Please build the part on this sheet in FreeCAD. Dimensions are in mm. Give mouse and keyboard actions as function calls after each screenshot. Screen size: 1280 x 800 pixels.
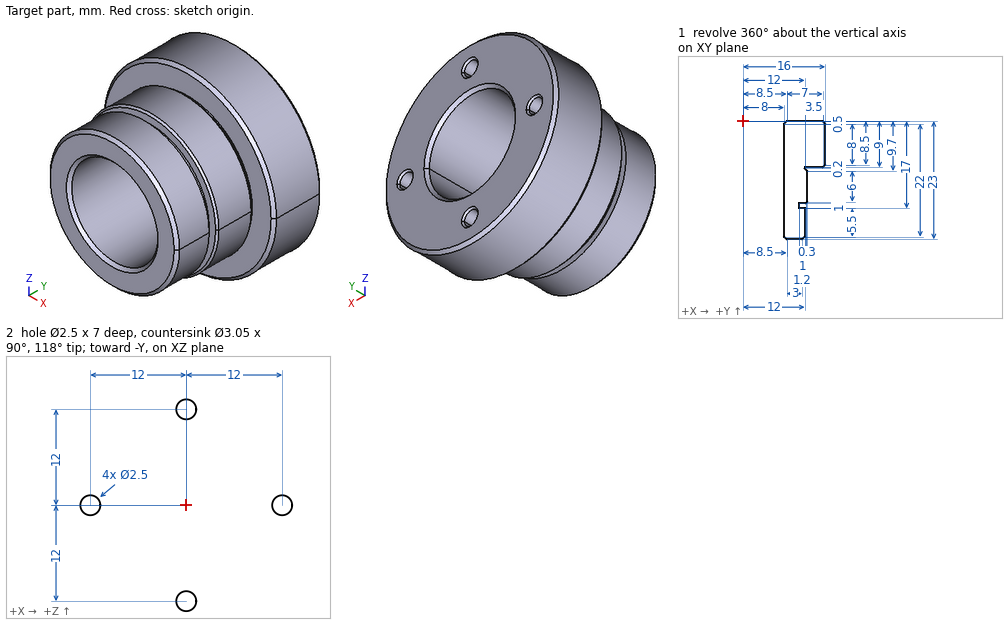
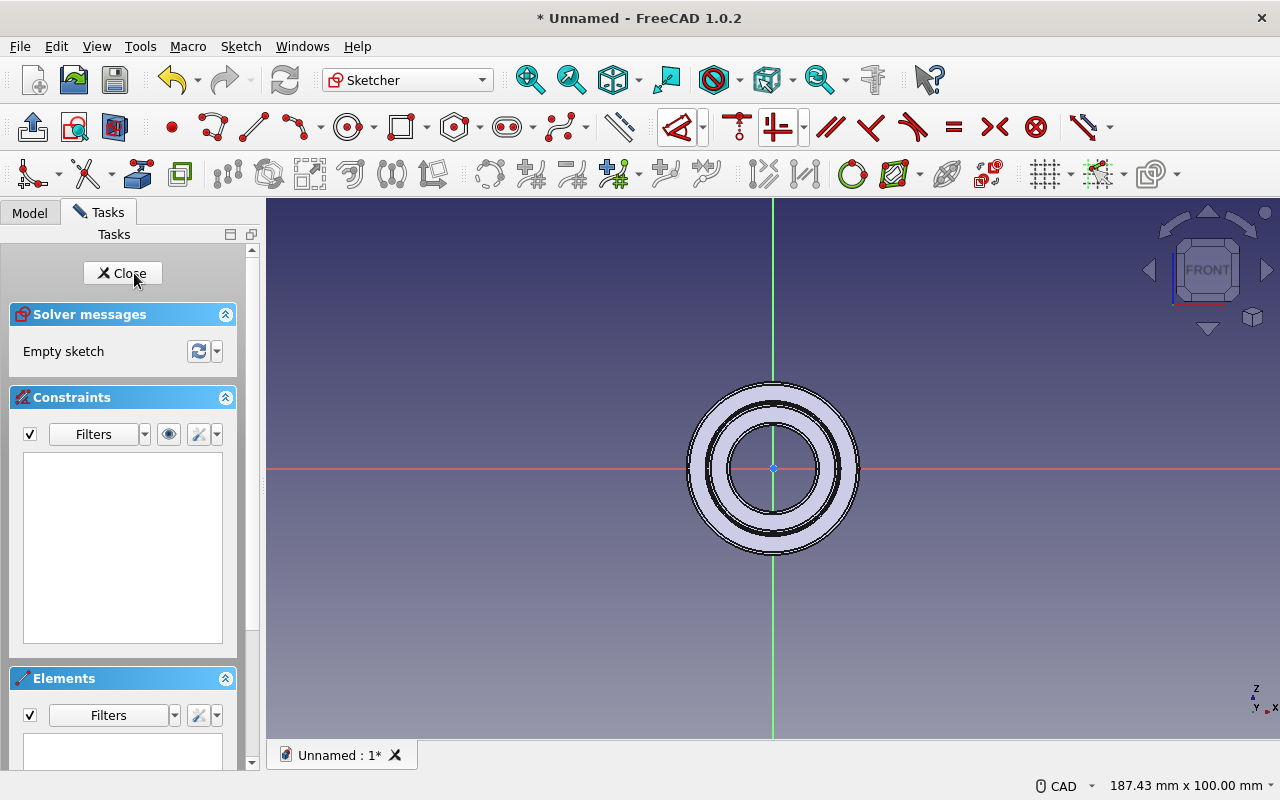
click(115, 128)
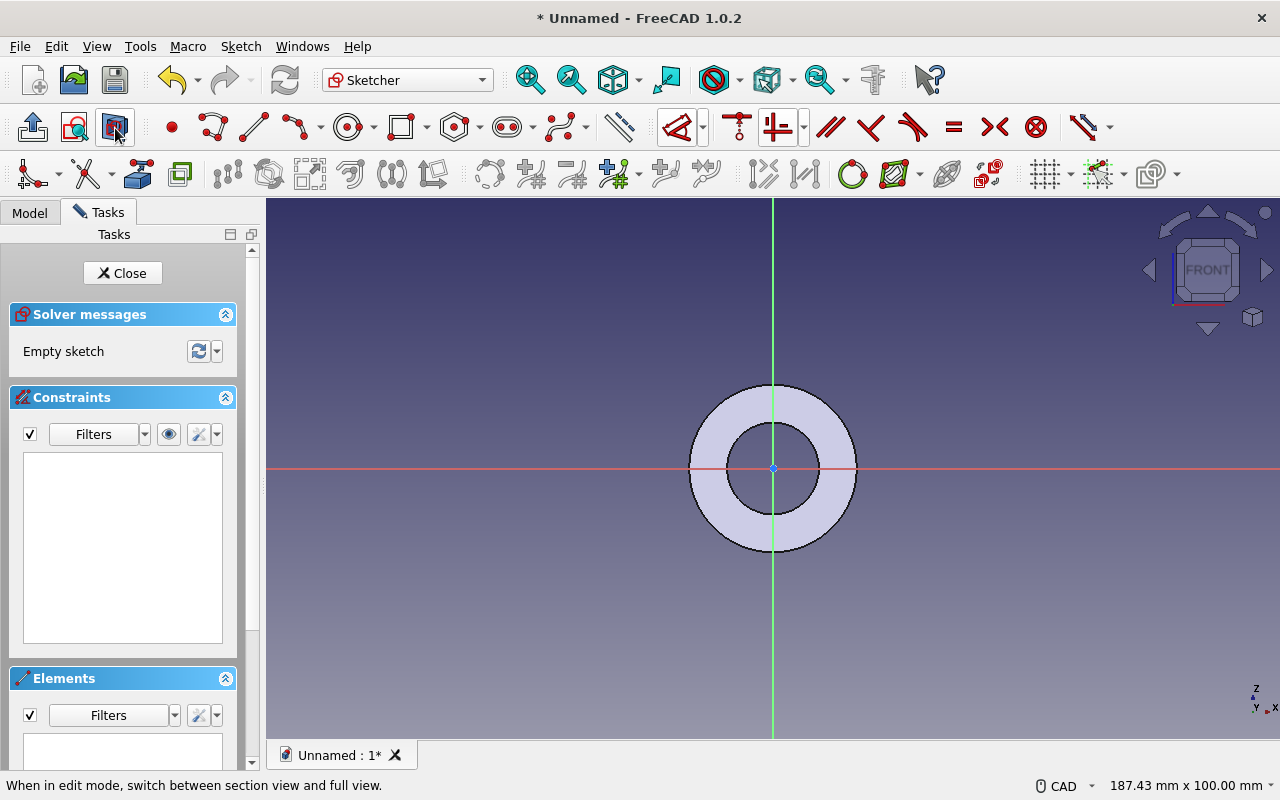
scroll(829, 469, up, 4)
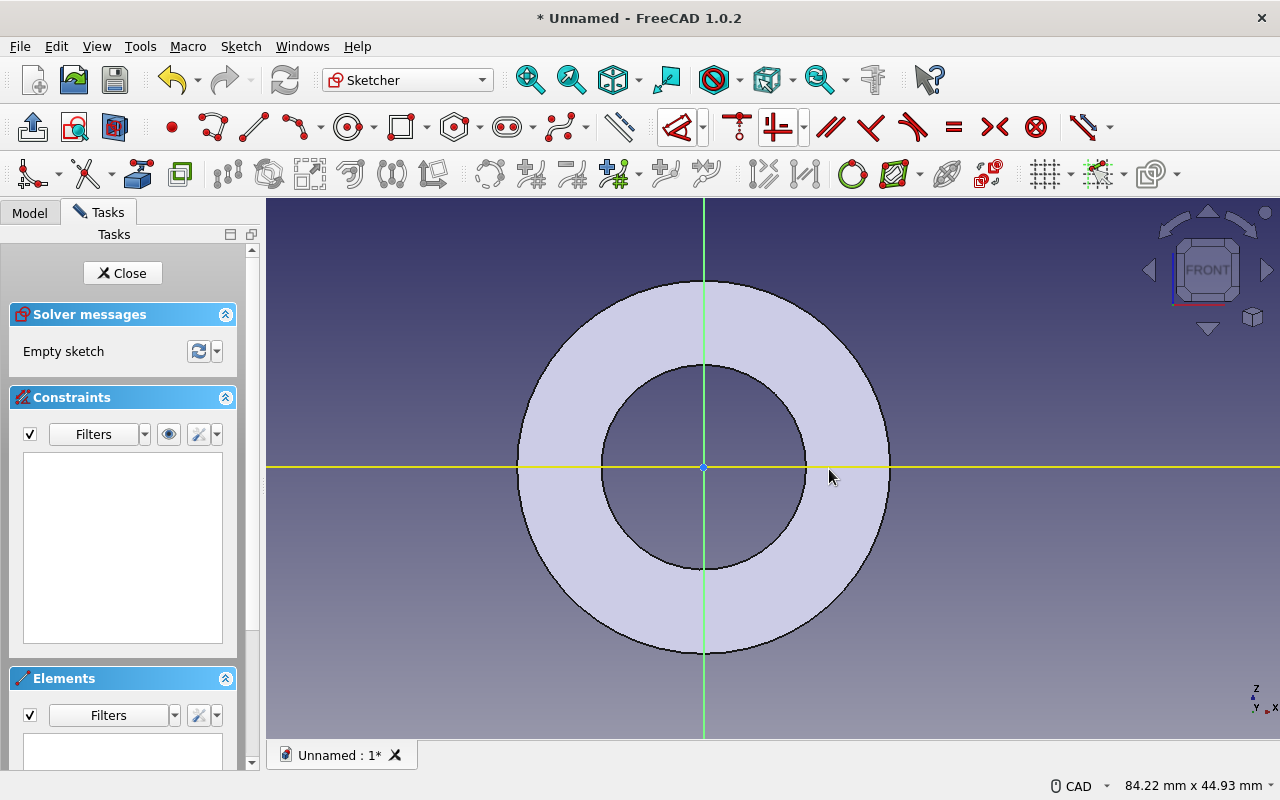
click(348, 128)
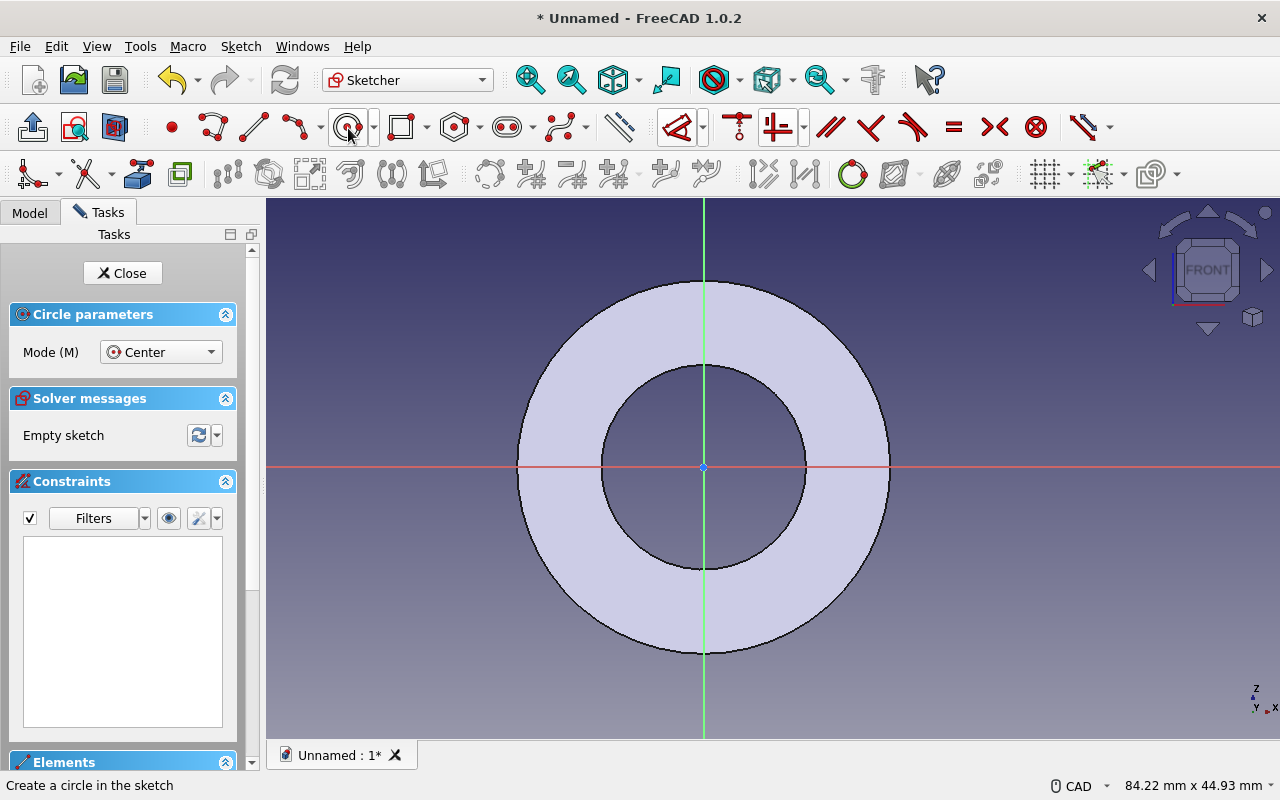
scroll(559, 467, up, 3)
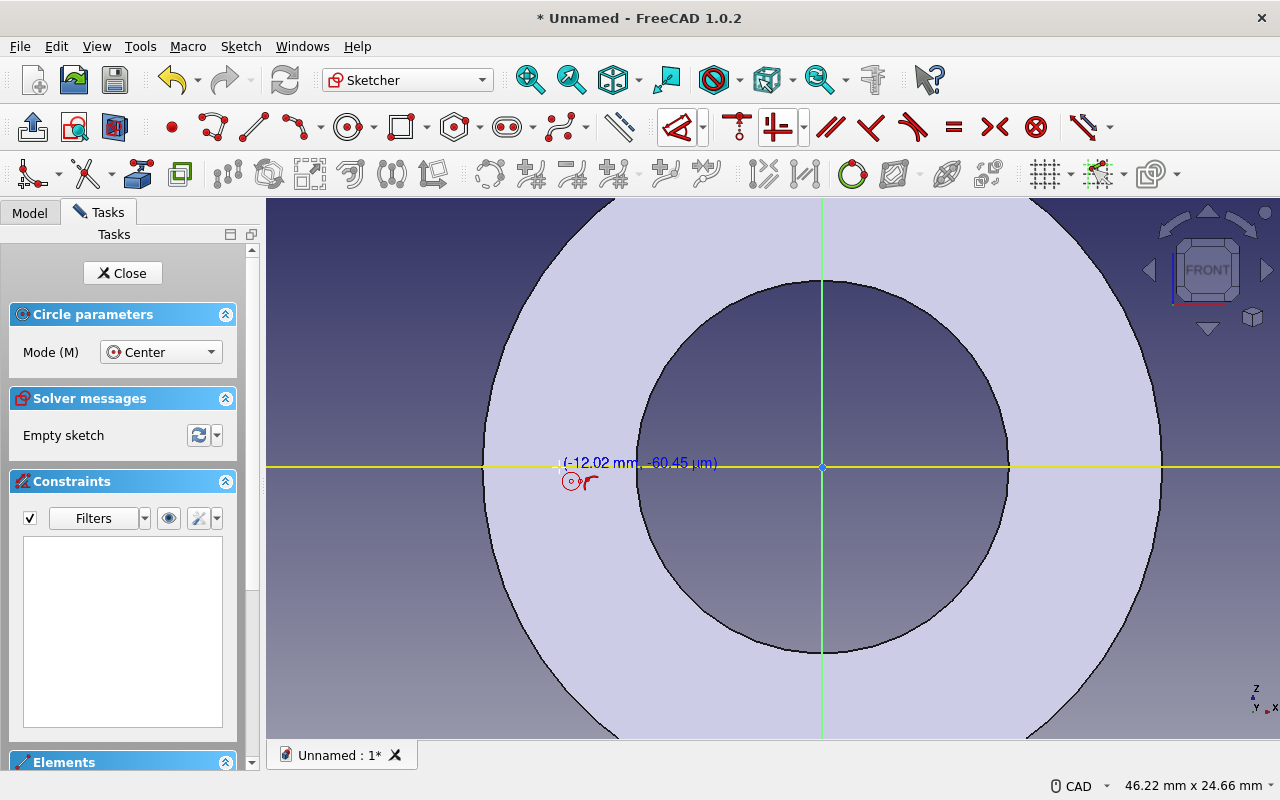
click(559, 467)
click(579, 448)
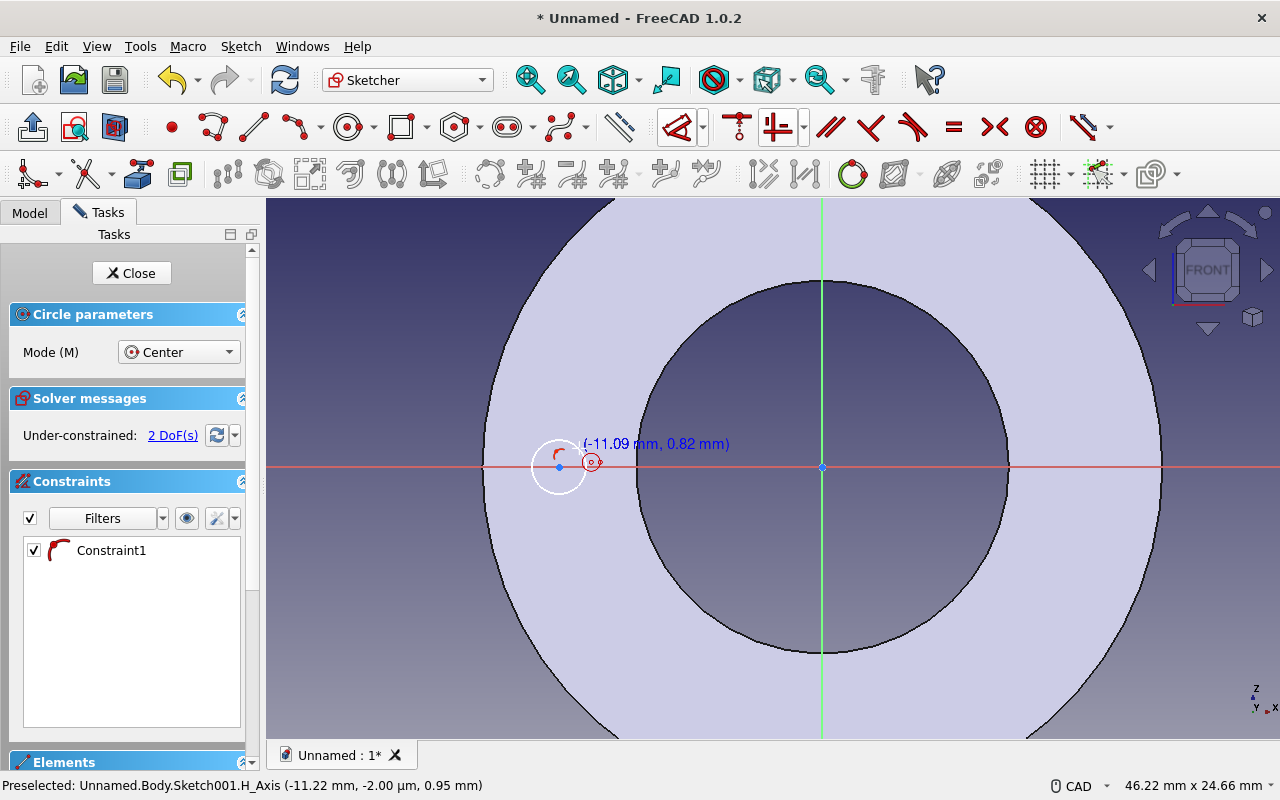
scroll(561, 470, down, 3)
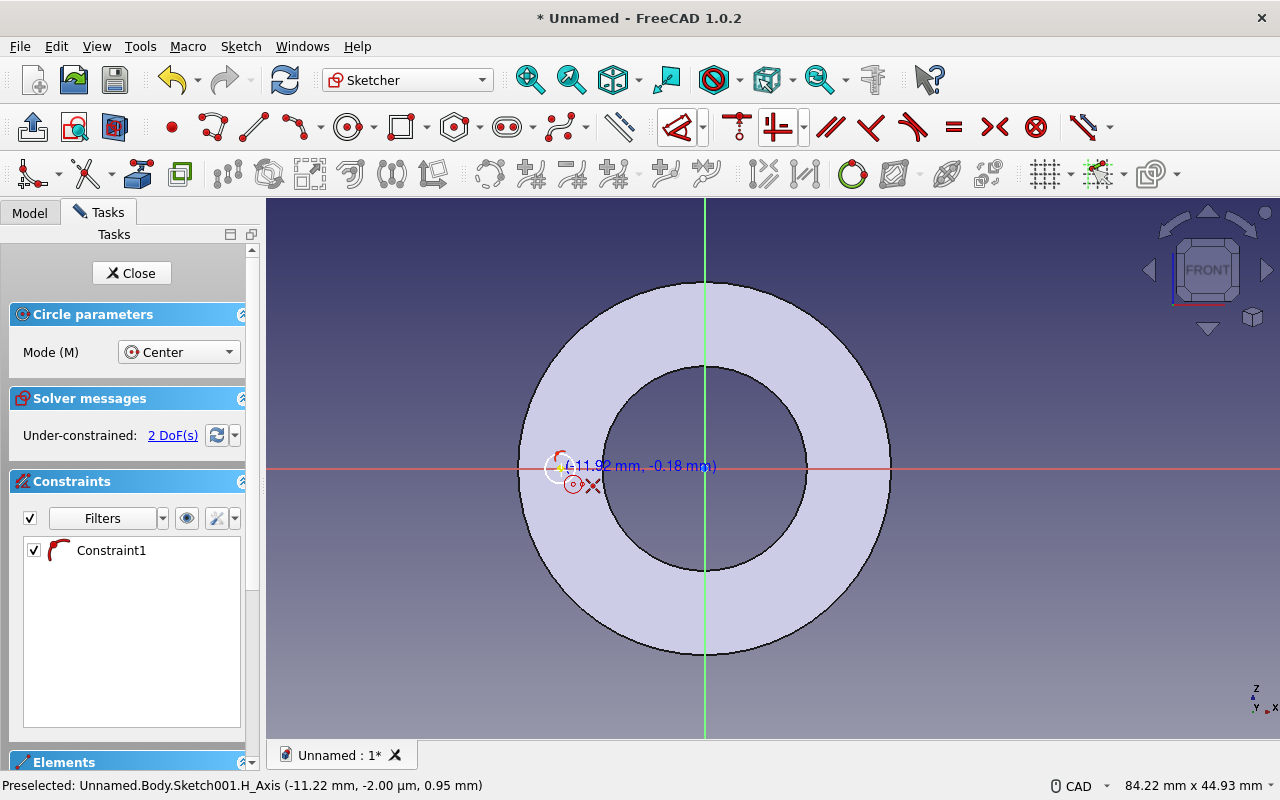
scroll(705, 613, up, 3)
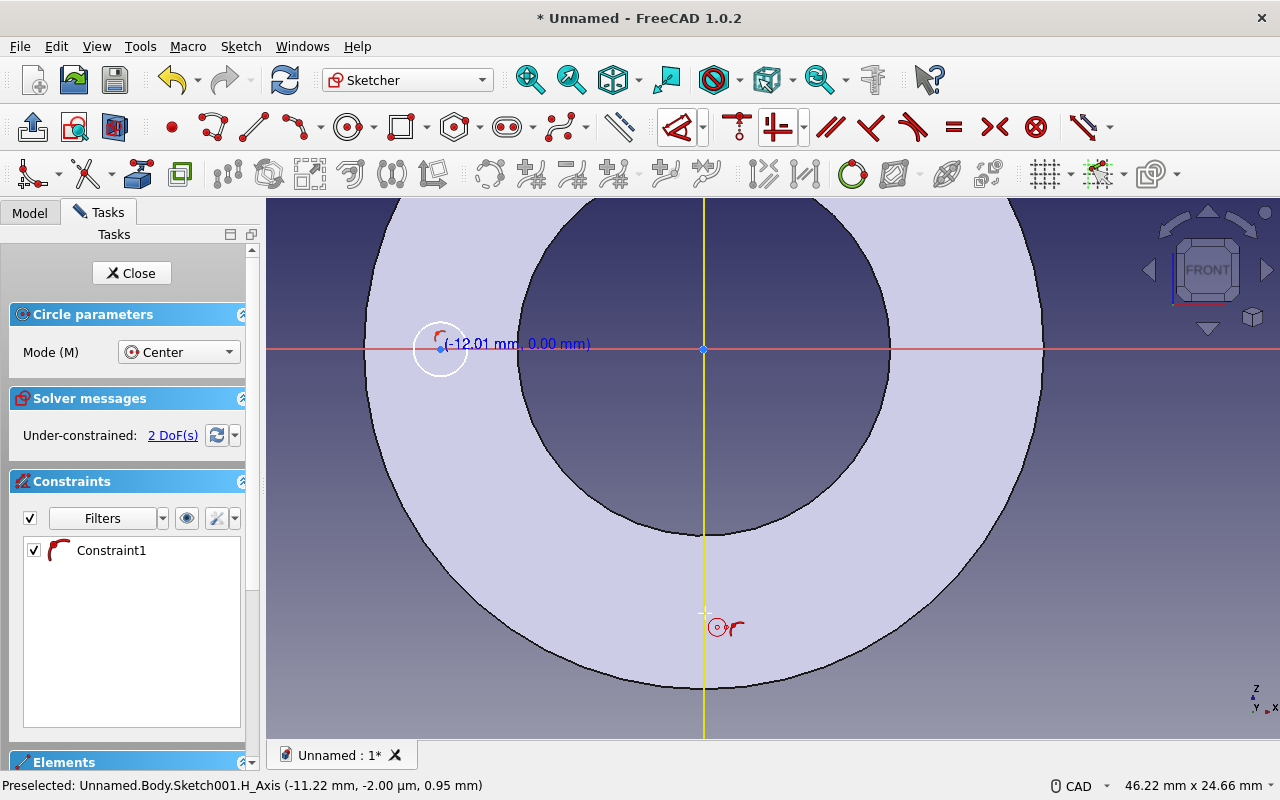
click(704, 613)
click(723, 593)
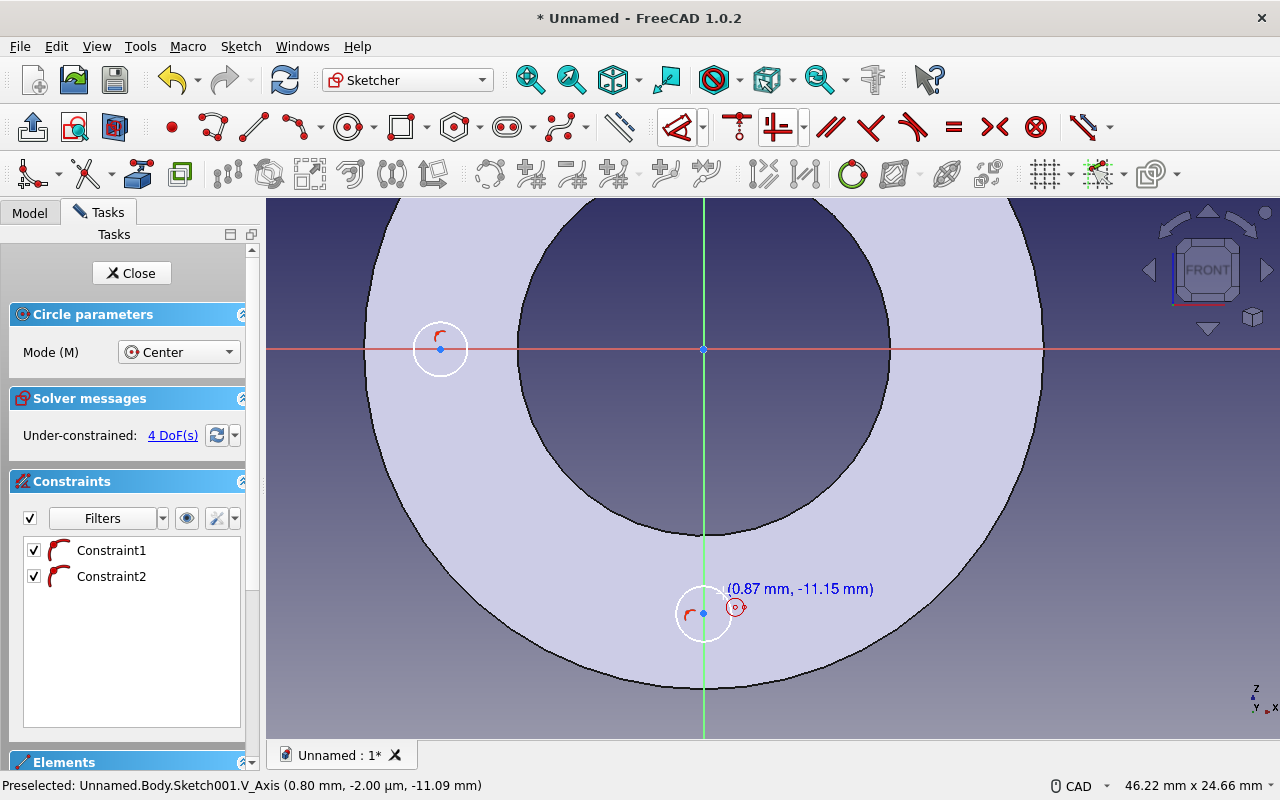
click(967, 349)
click(987, 330)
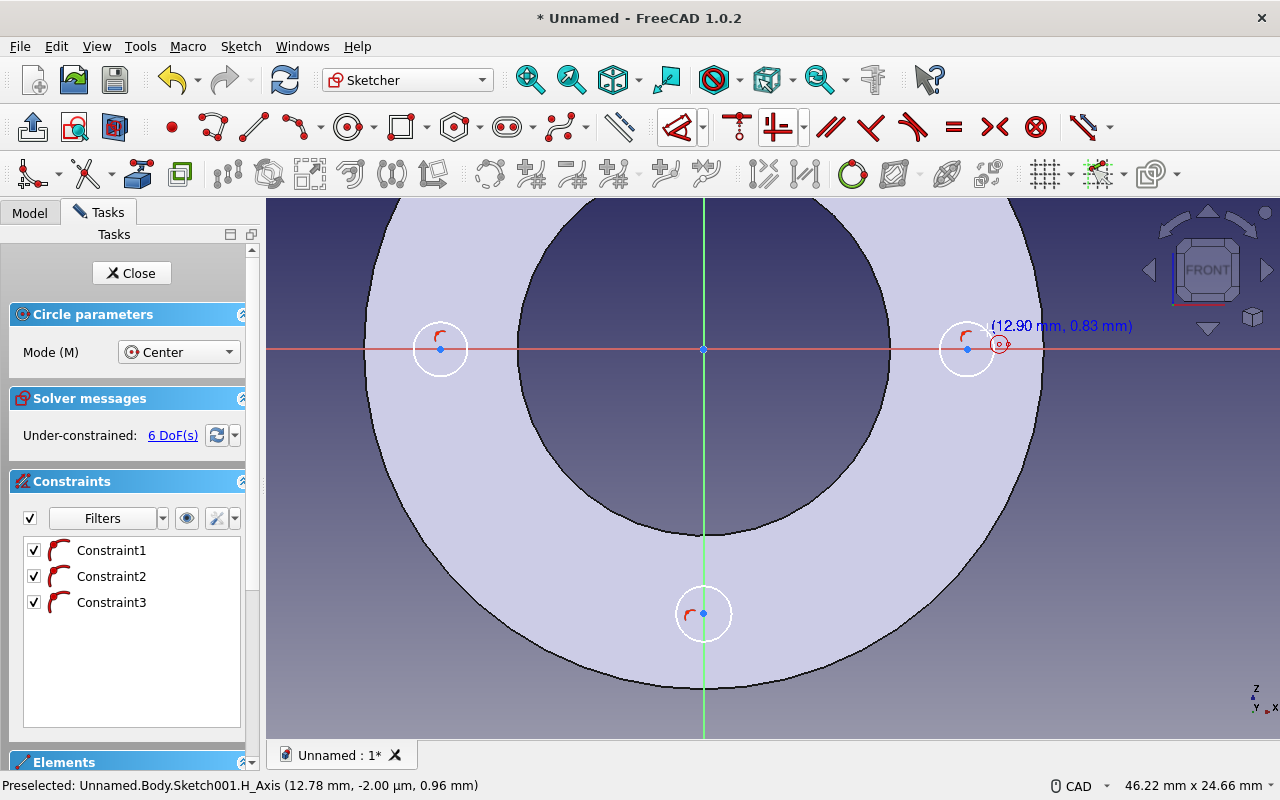
scroll(705, 613, down, 3)